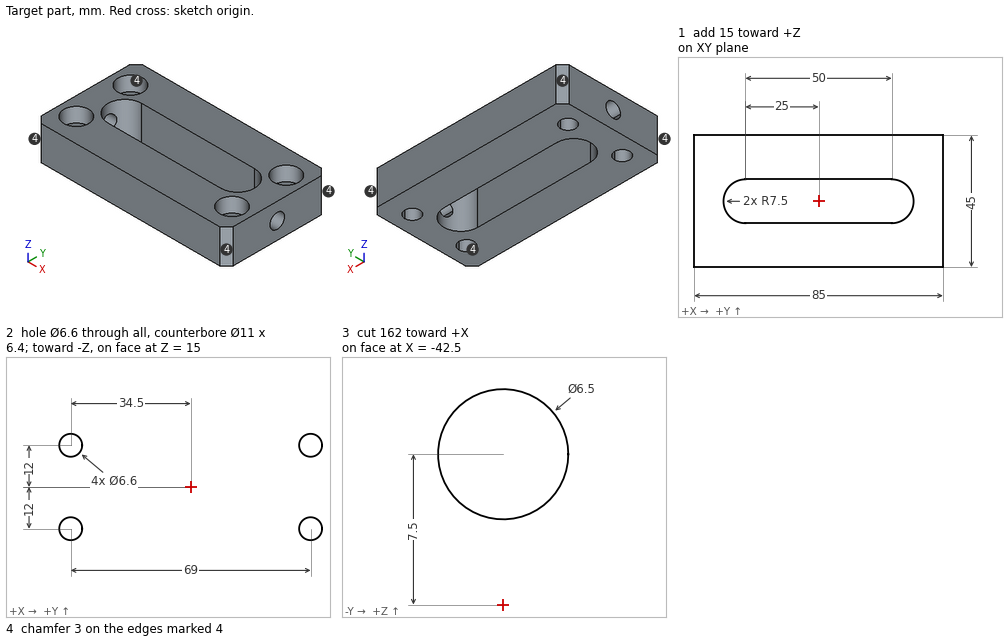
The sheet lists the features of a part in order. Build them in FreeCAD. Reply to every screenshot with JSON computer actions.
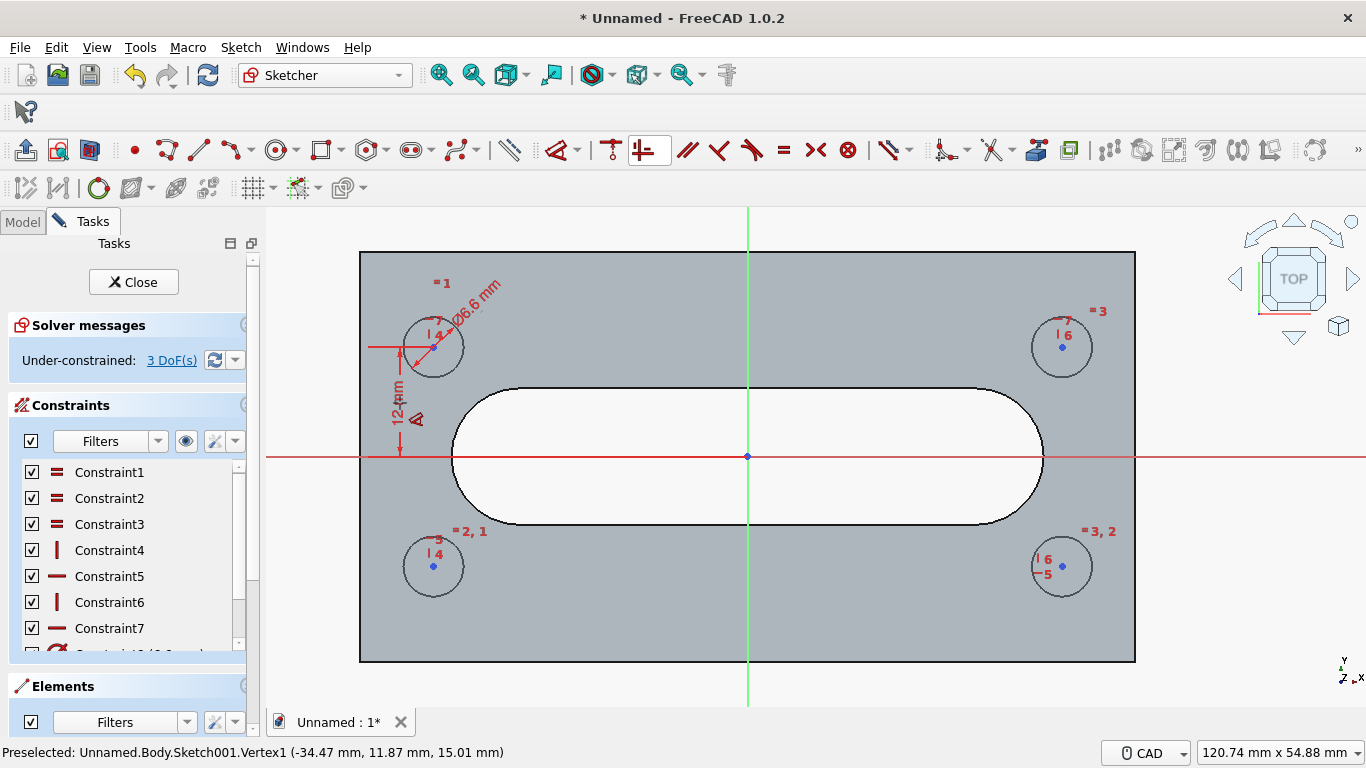
{"action": "left_click", "coordinate": [434, 567]}
{"action": "left_click", "coordinate": [400, 512]}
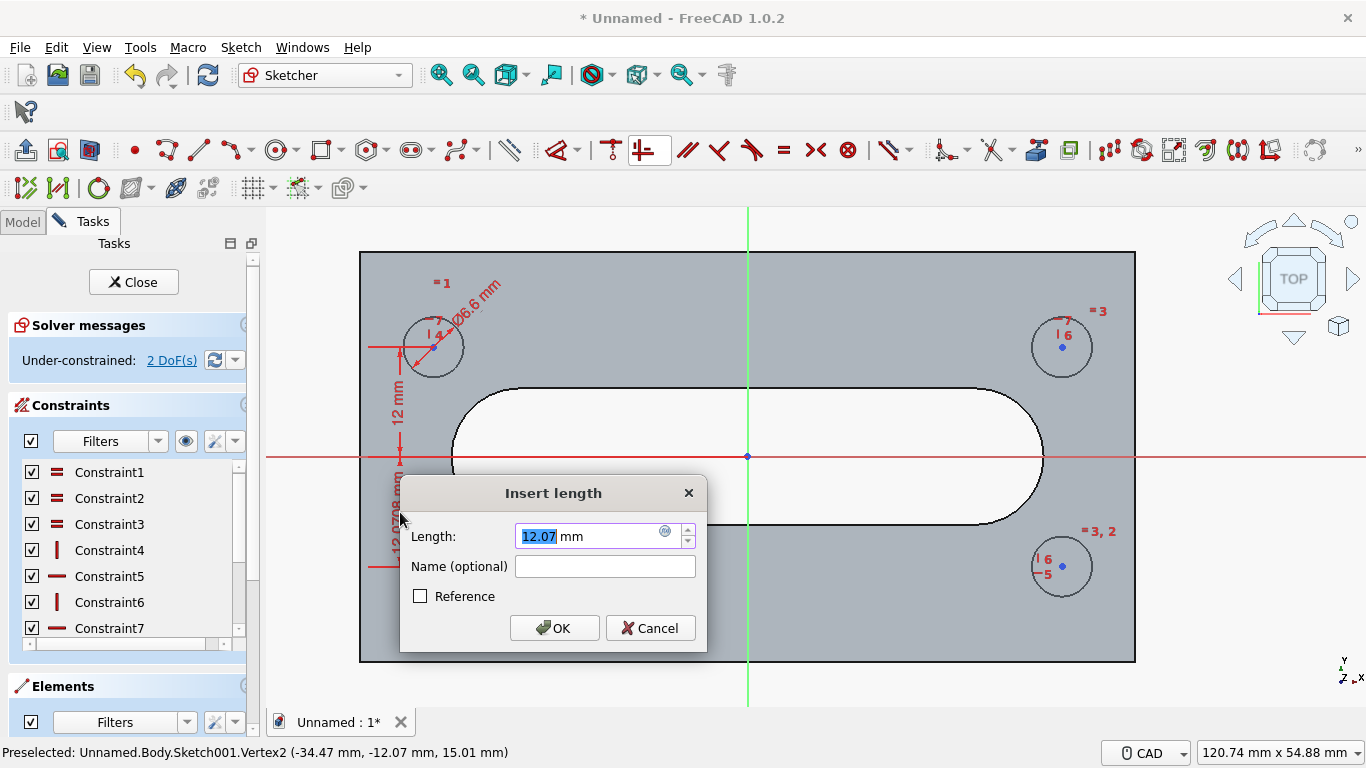
{"action": "type", "text": "12"}
{"action": "key", "text": "Return"}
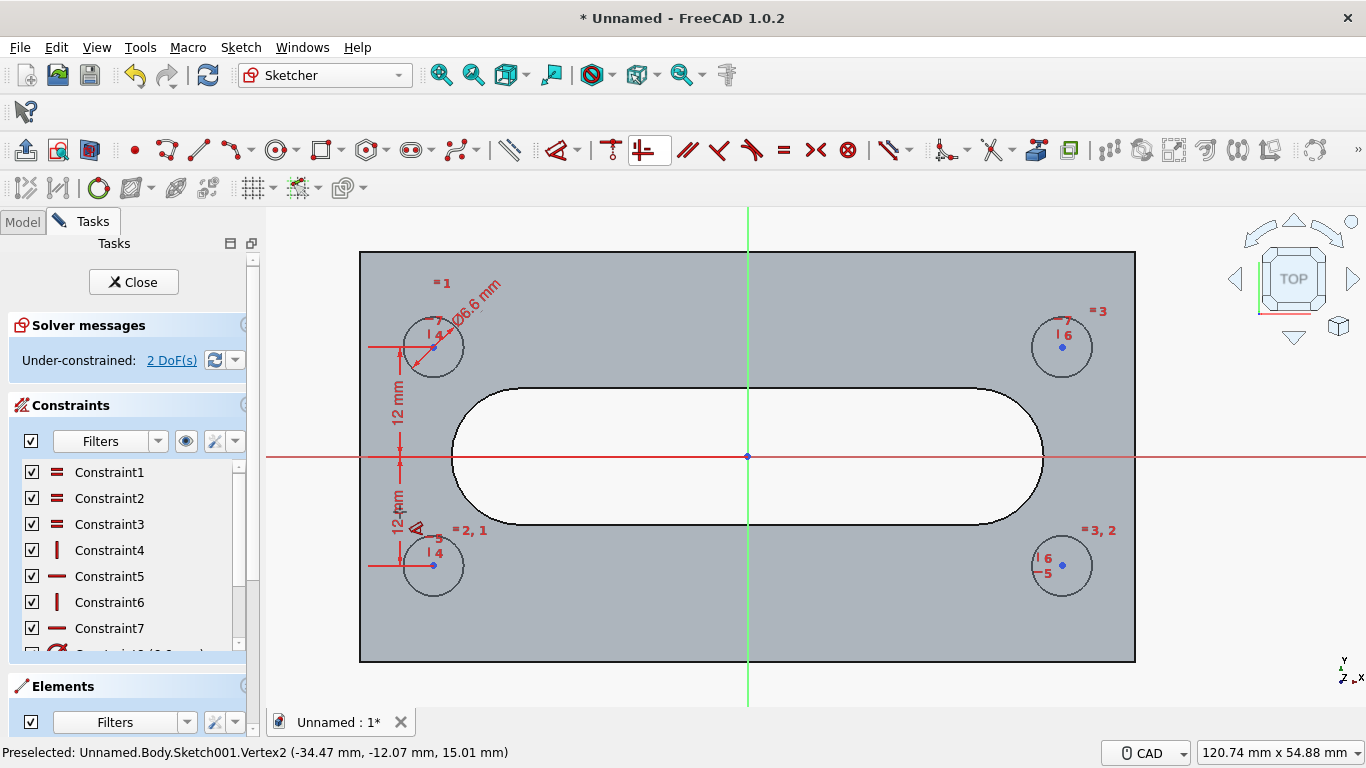
{"action": "left_click", "coordinate": [434, 566]}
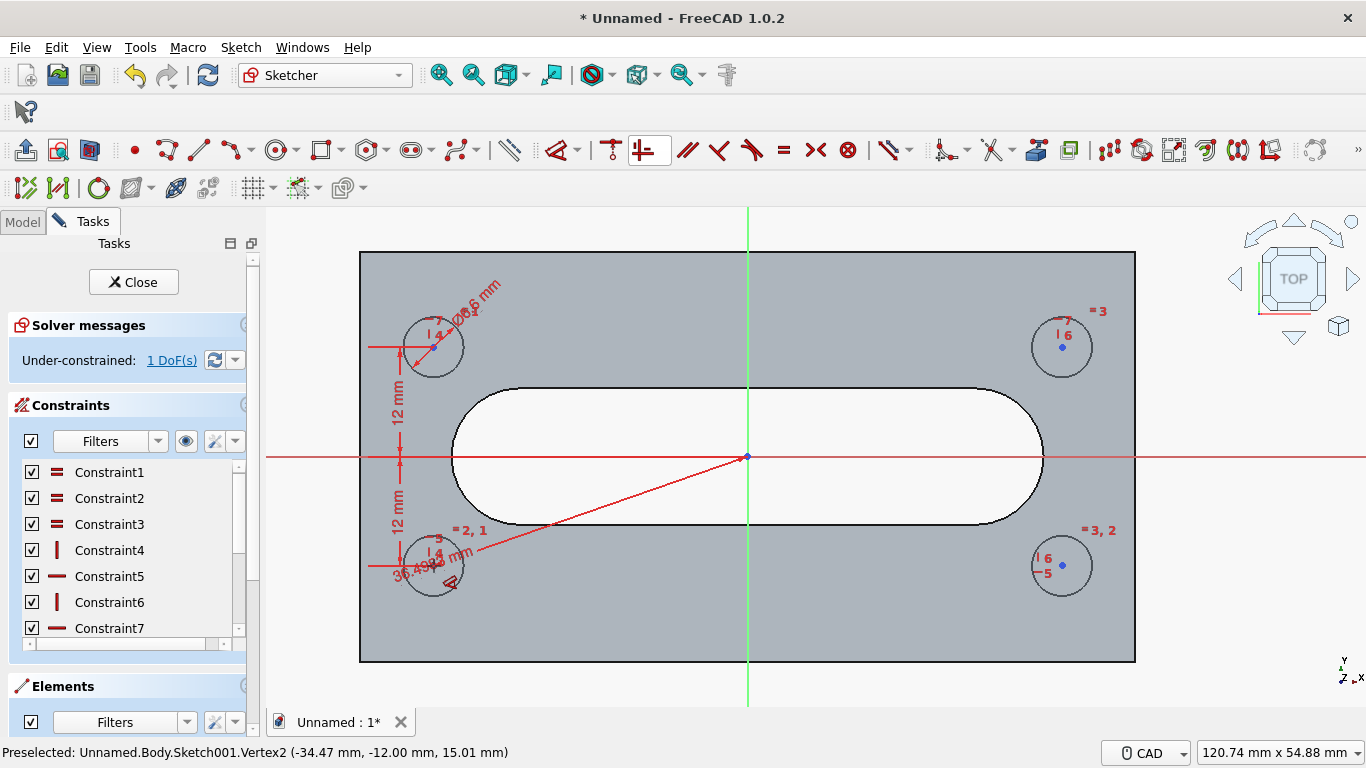
{"action": "left_click", "coordinate": [1062, 566]}
{"action": "left_click", "coordinate": [603, 600]}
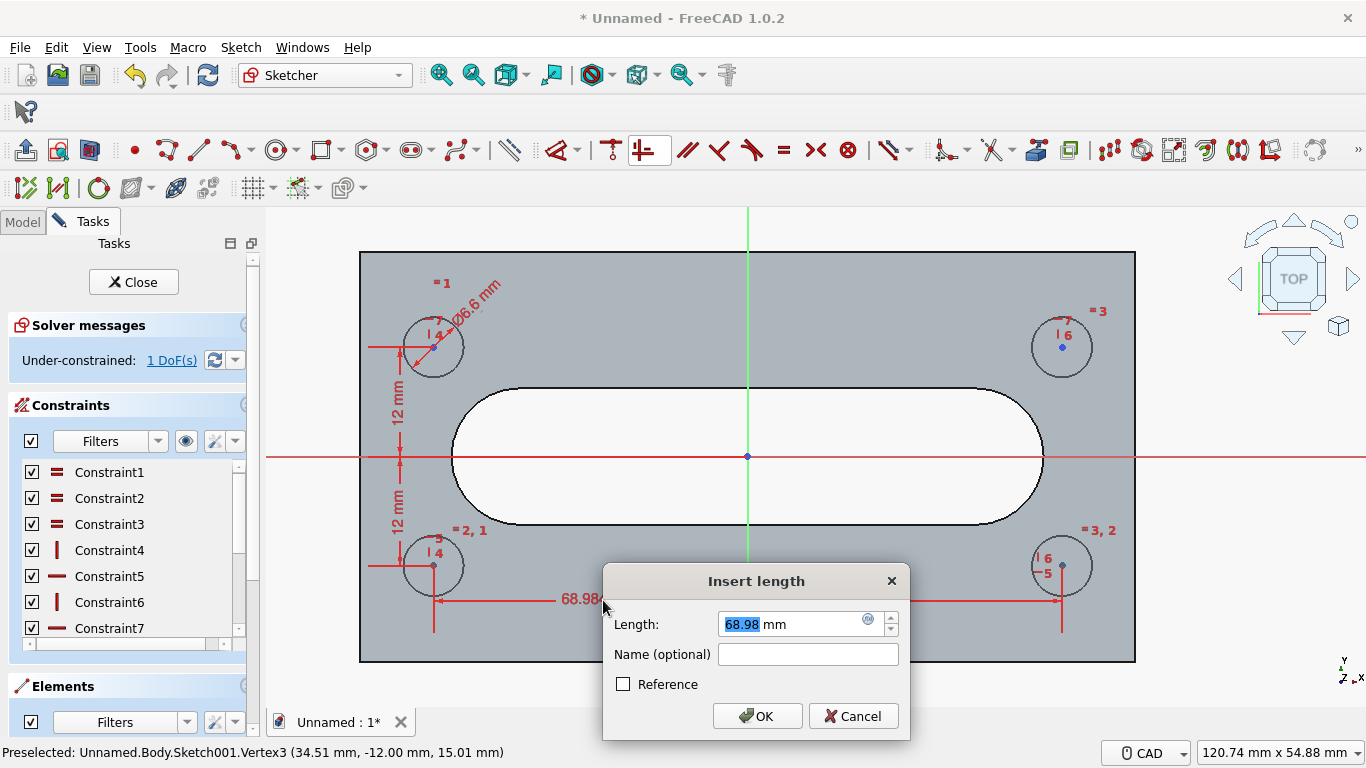
{"action": "type", "text": "69"}
{"action": "key", "text": "Return"}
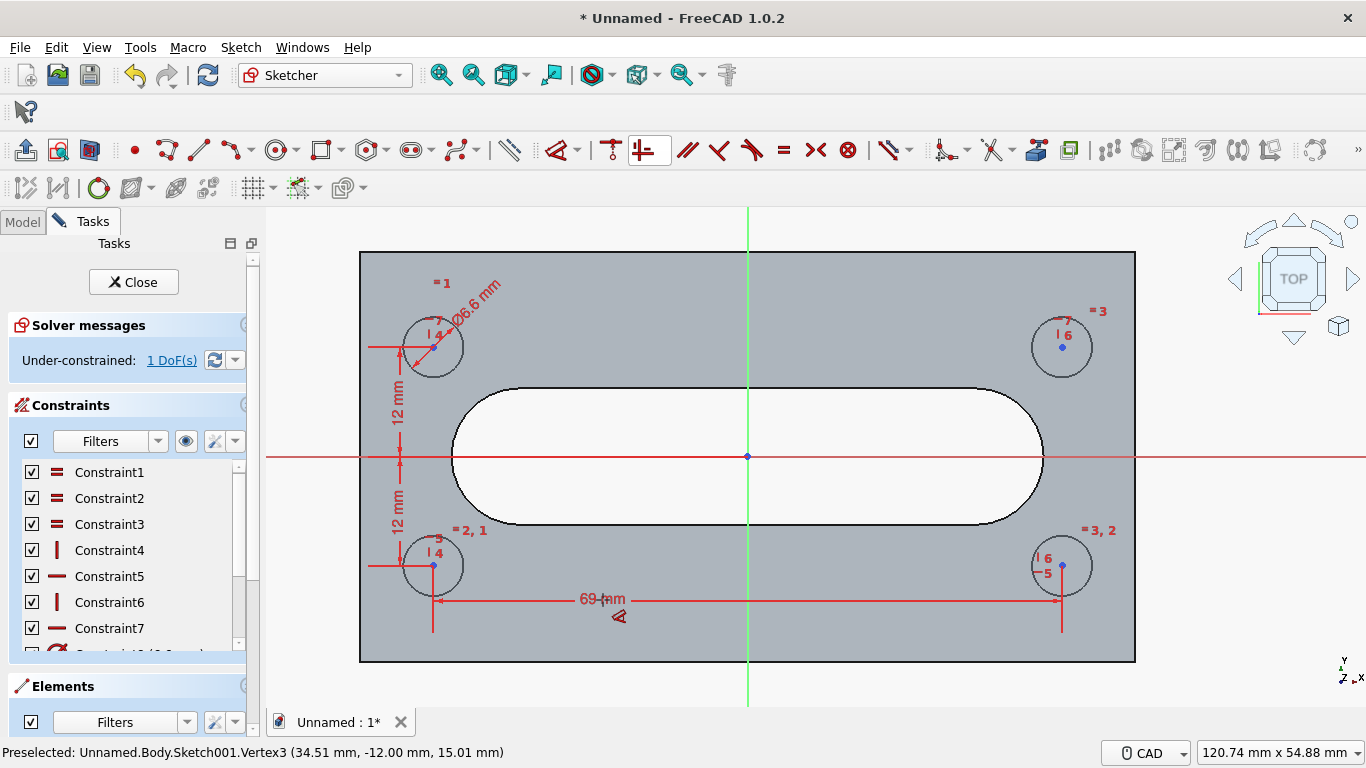
{"action": "left_click", "coordinate": [433, 347]}
{"action": "left_click", "coordinate": [590, 313]}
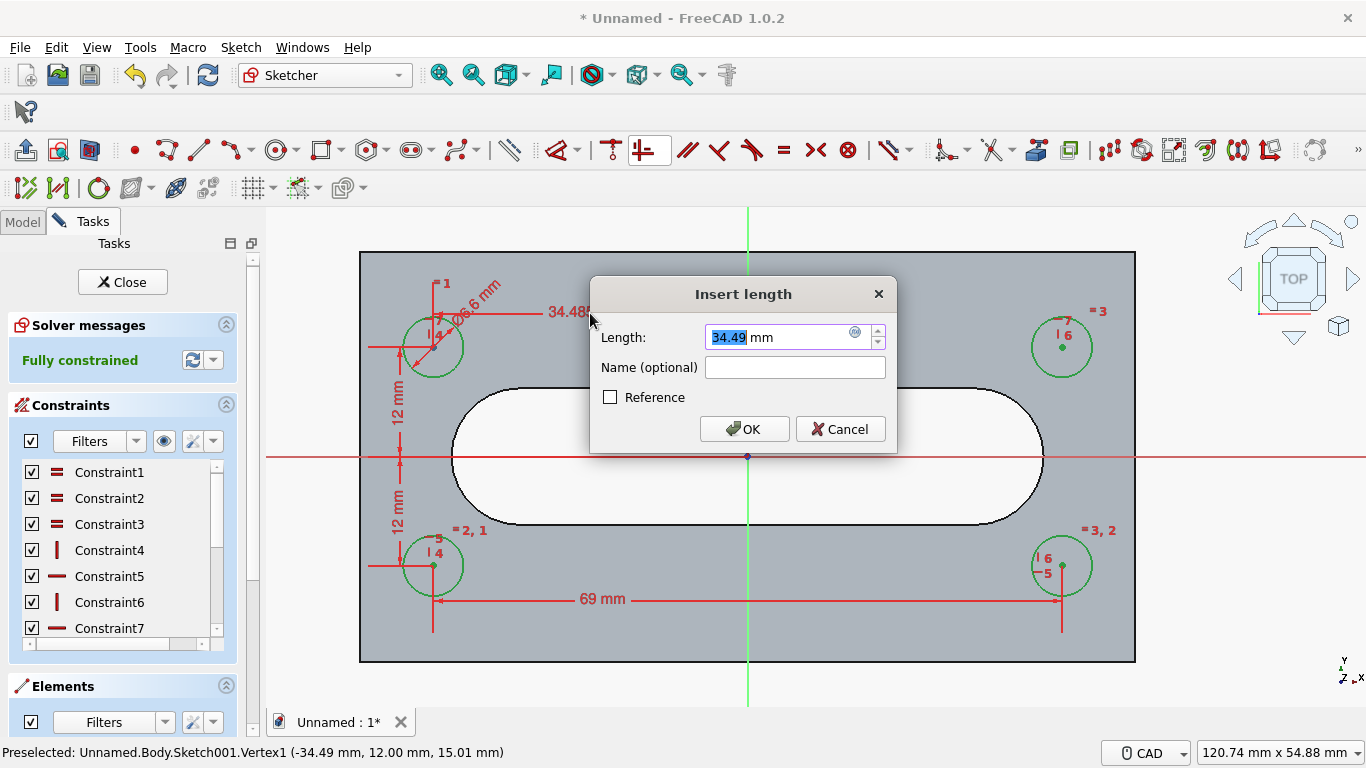
{"action": "type", "text": "34.5"}
{"action": "key", "text": "Return"}
{"action": "key", "text": "Escape"}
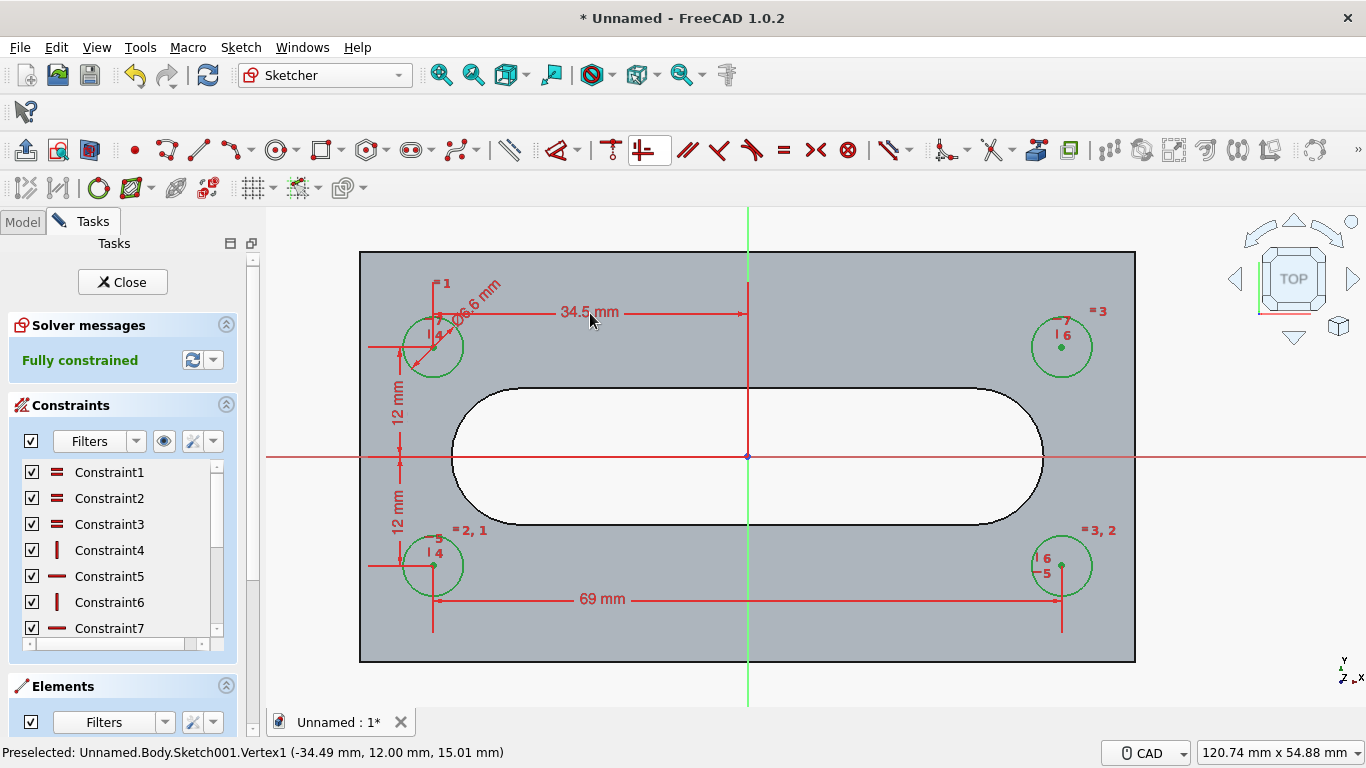
{"action": "left_click", "coordinate": [123, 282]}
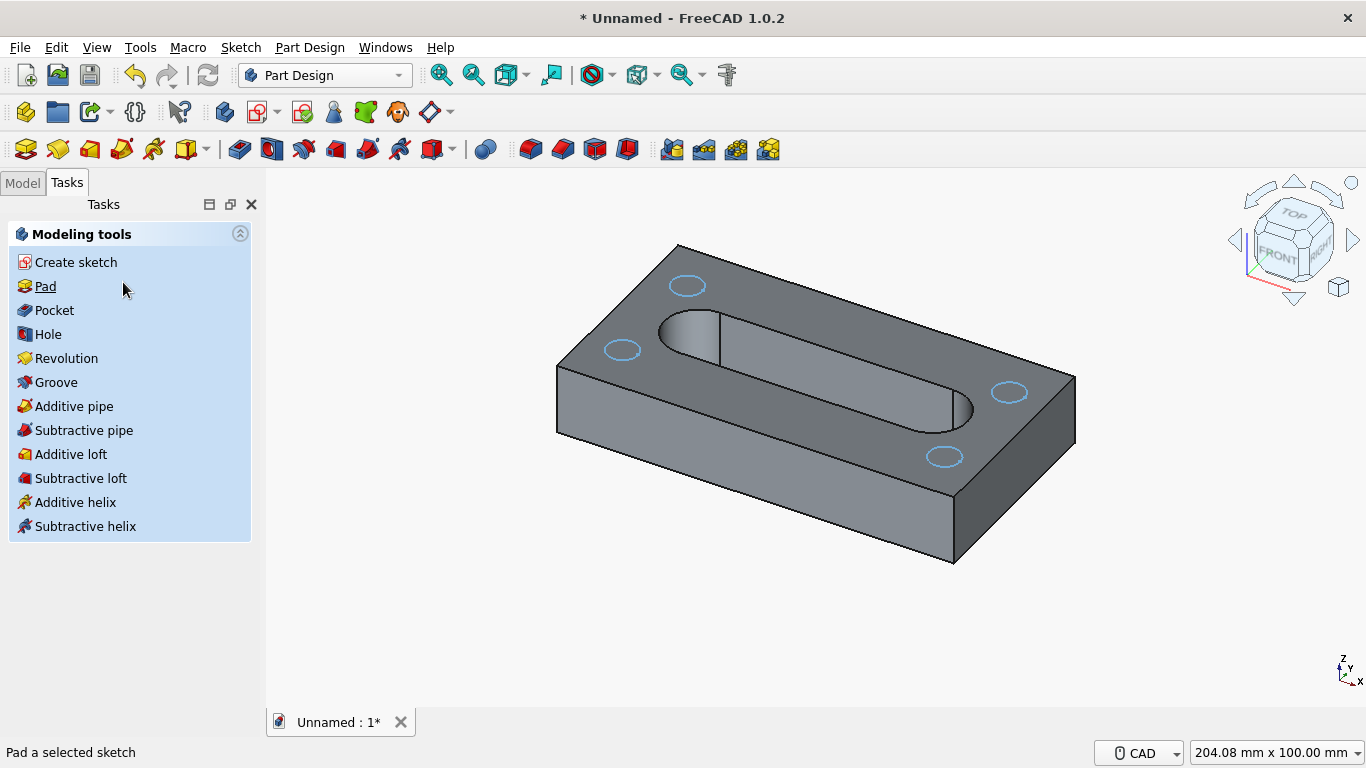
{"action": "left_click", "coordinate": [272, 150]}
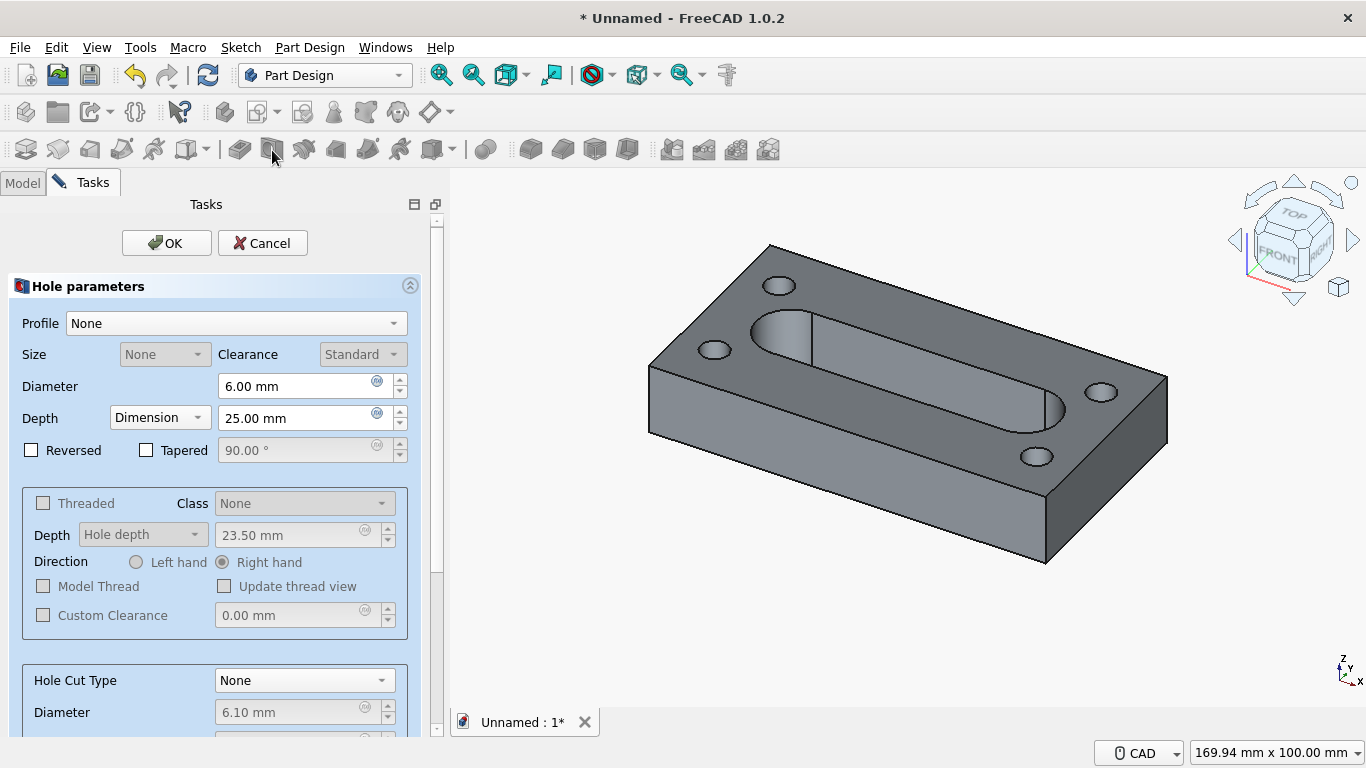
{"action": "triple_click", "coordinate": [305, 386]}